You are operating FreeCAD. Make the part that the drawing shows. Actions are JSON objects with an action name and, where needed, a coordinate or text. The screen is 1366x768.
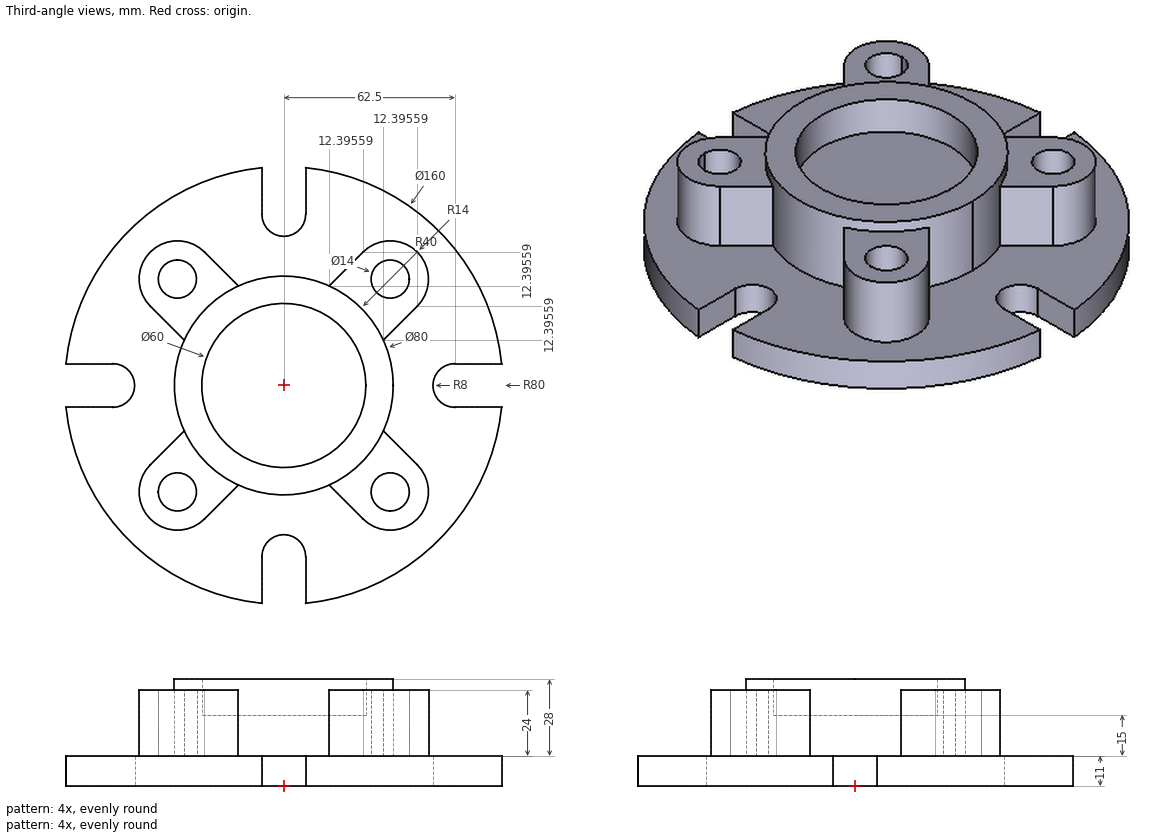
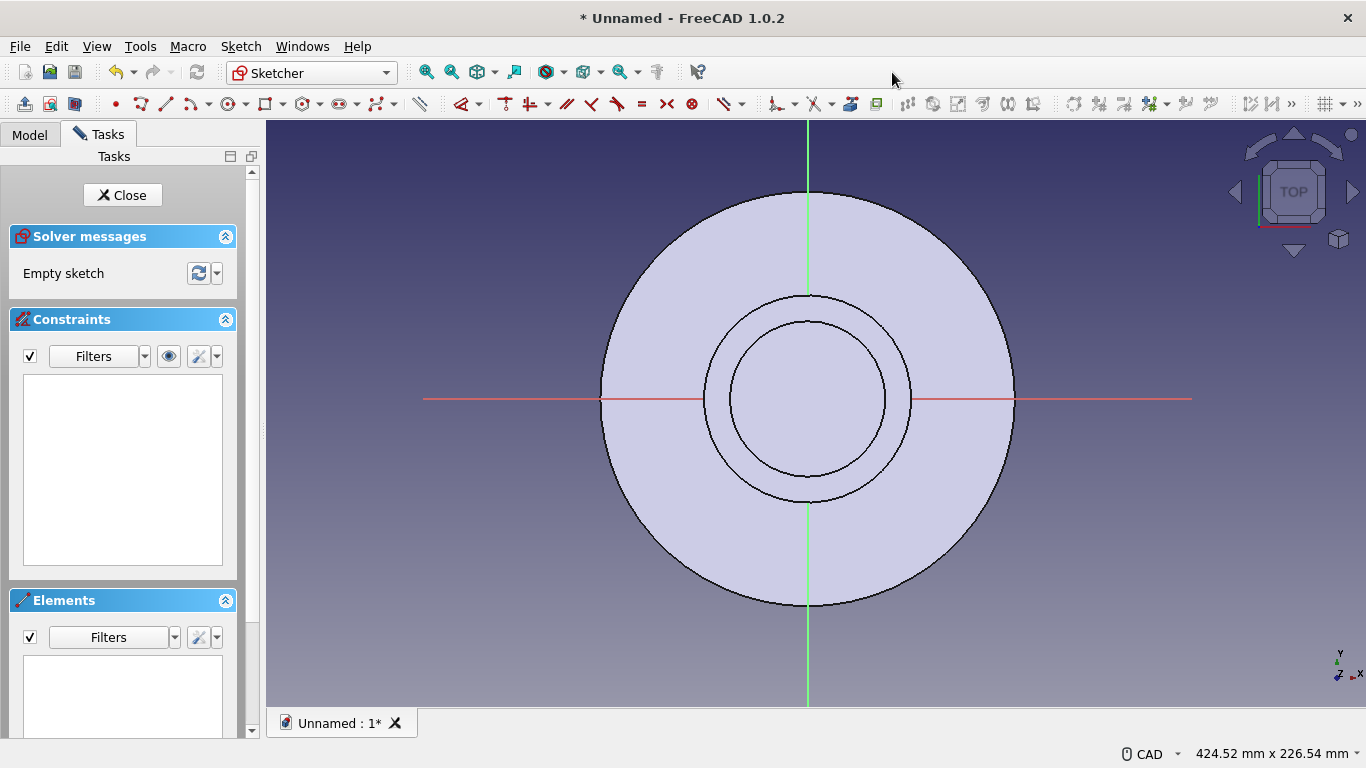
{"action": "key", "text": "q s"}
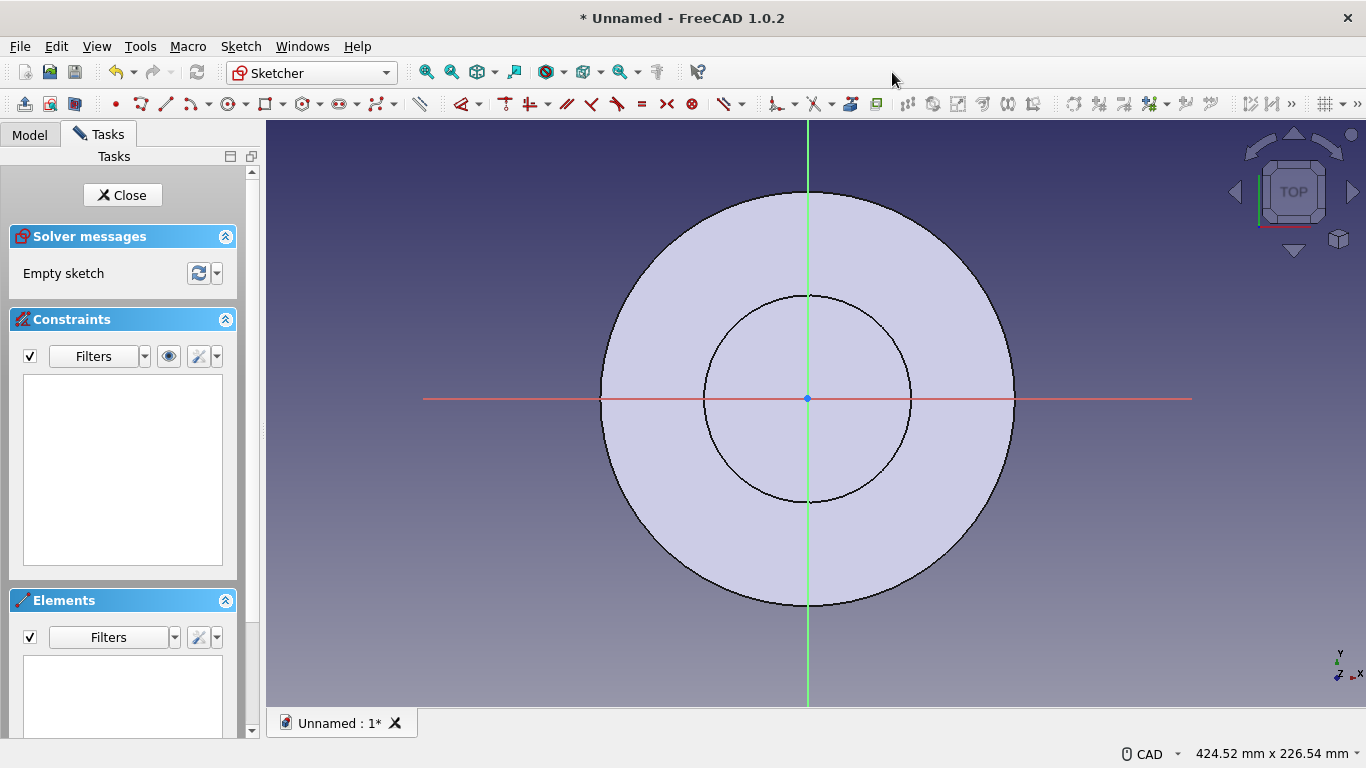
{"action": "scroll", "coordinate": [943, 291], "scroll_direction": "up", "scroll_amount": 5}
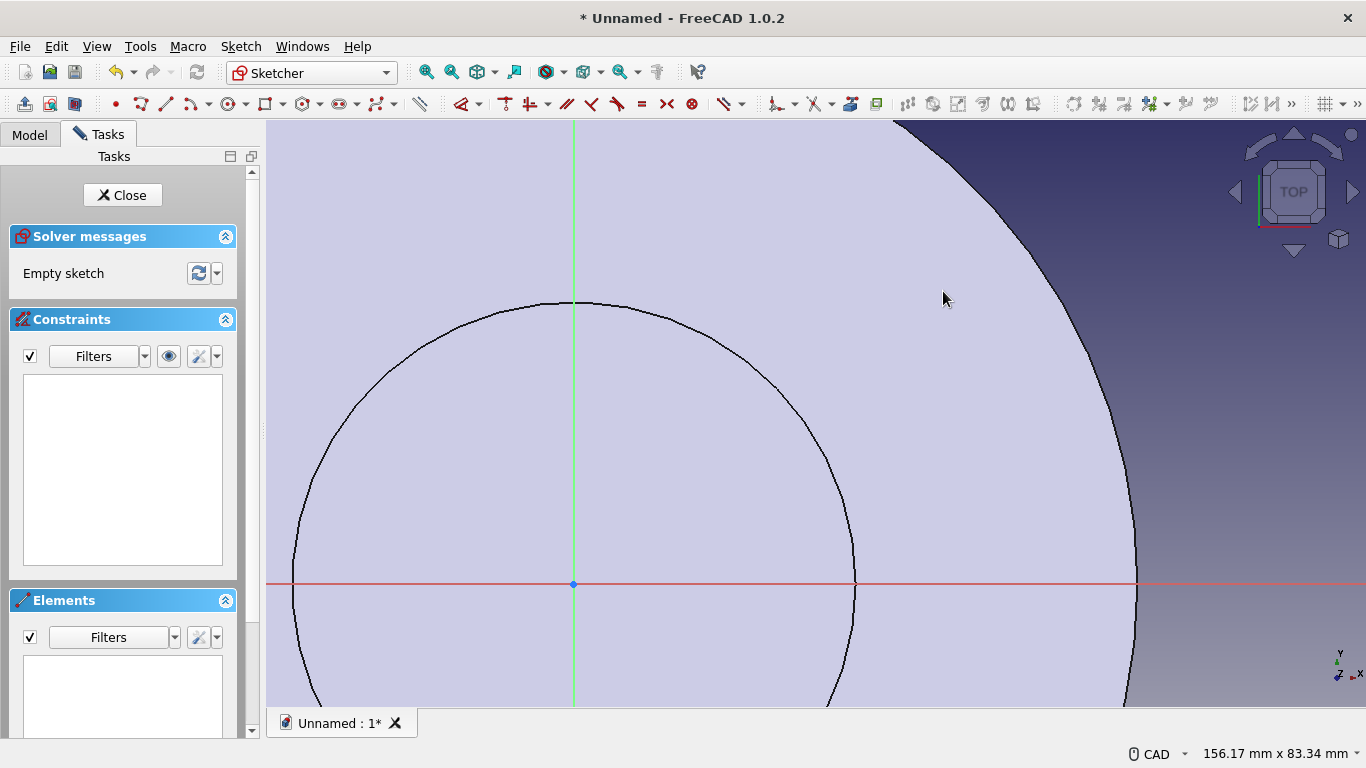
{"action": "key", "text": "g l"}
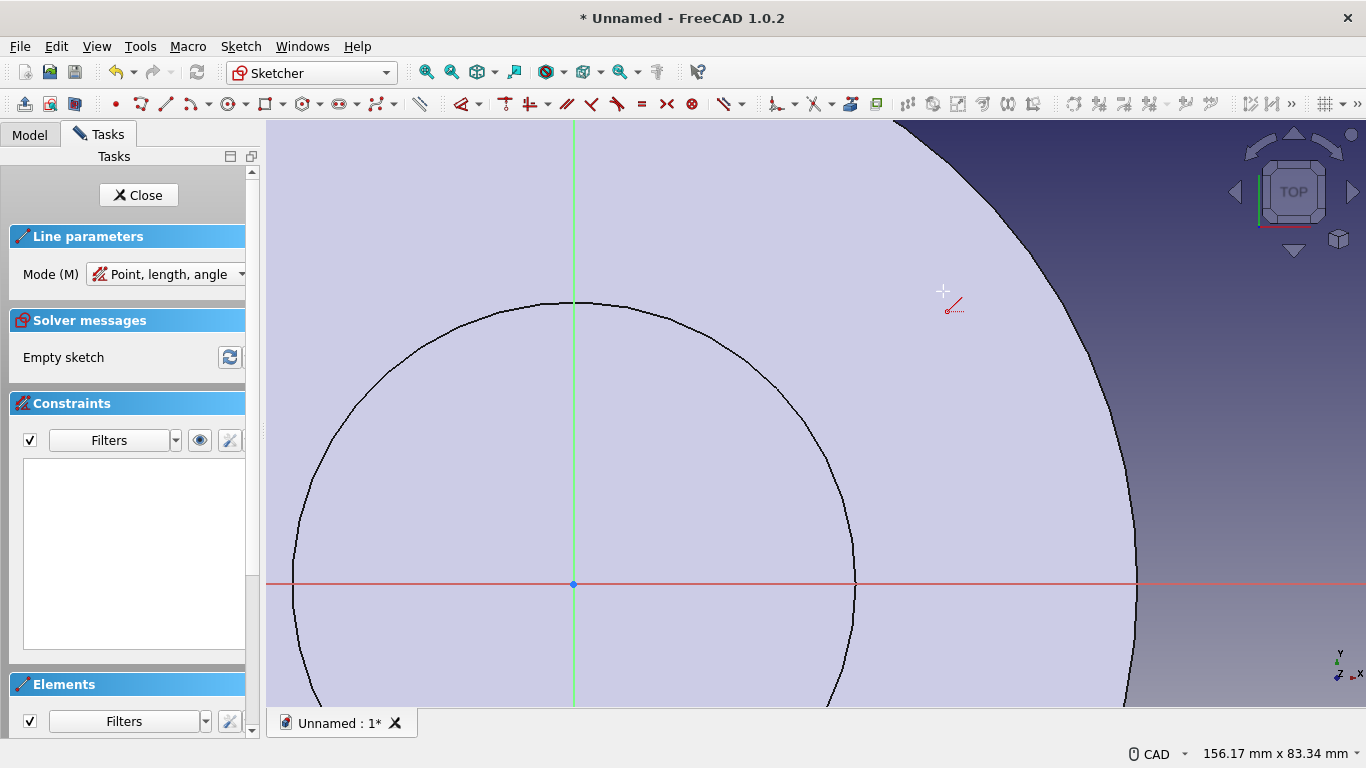
{"action": "left_click", "coordinate": [778, 240]}
{"action": "left_click", "coordinate": [691, 328]}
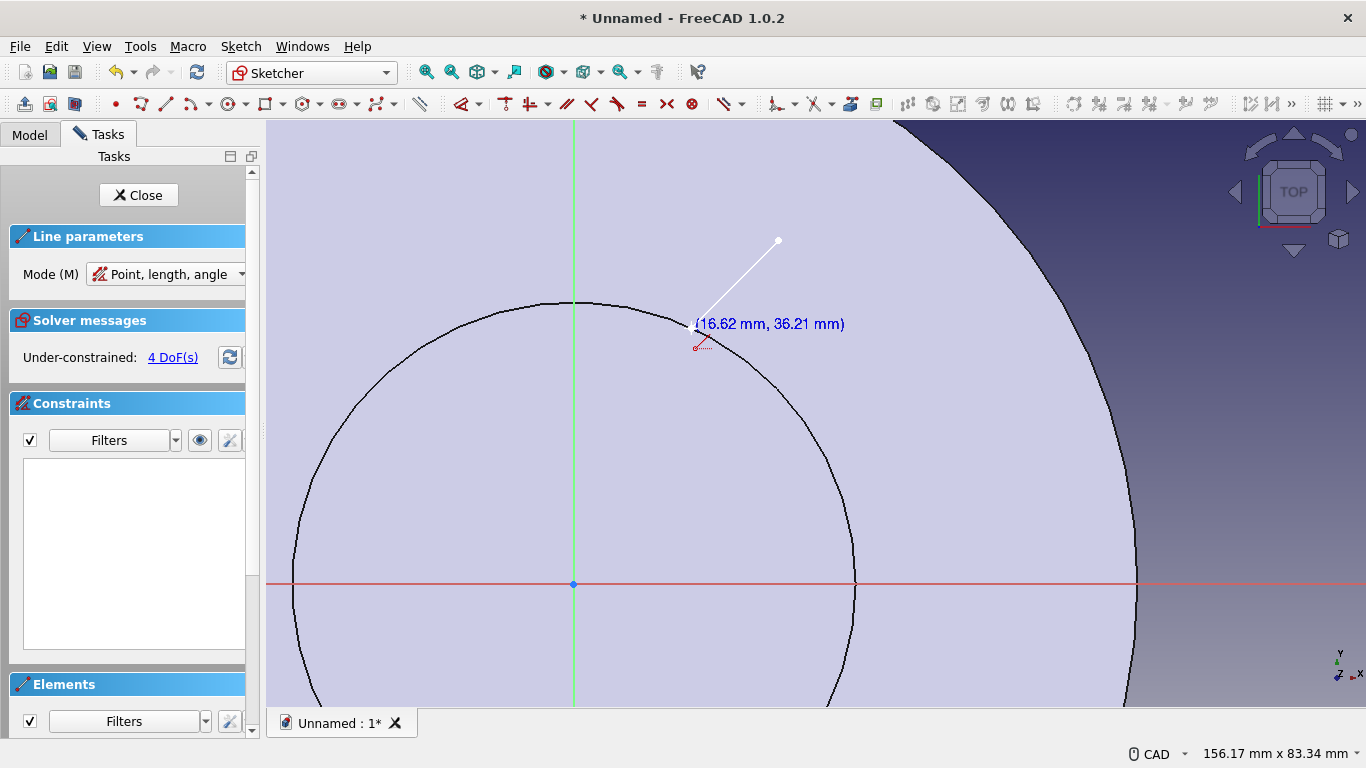
{"action": "left_click", "coordinate": [830, 467]}
{"action": "left_click", "coordinate": [918, 380]}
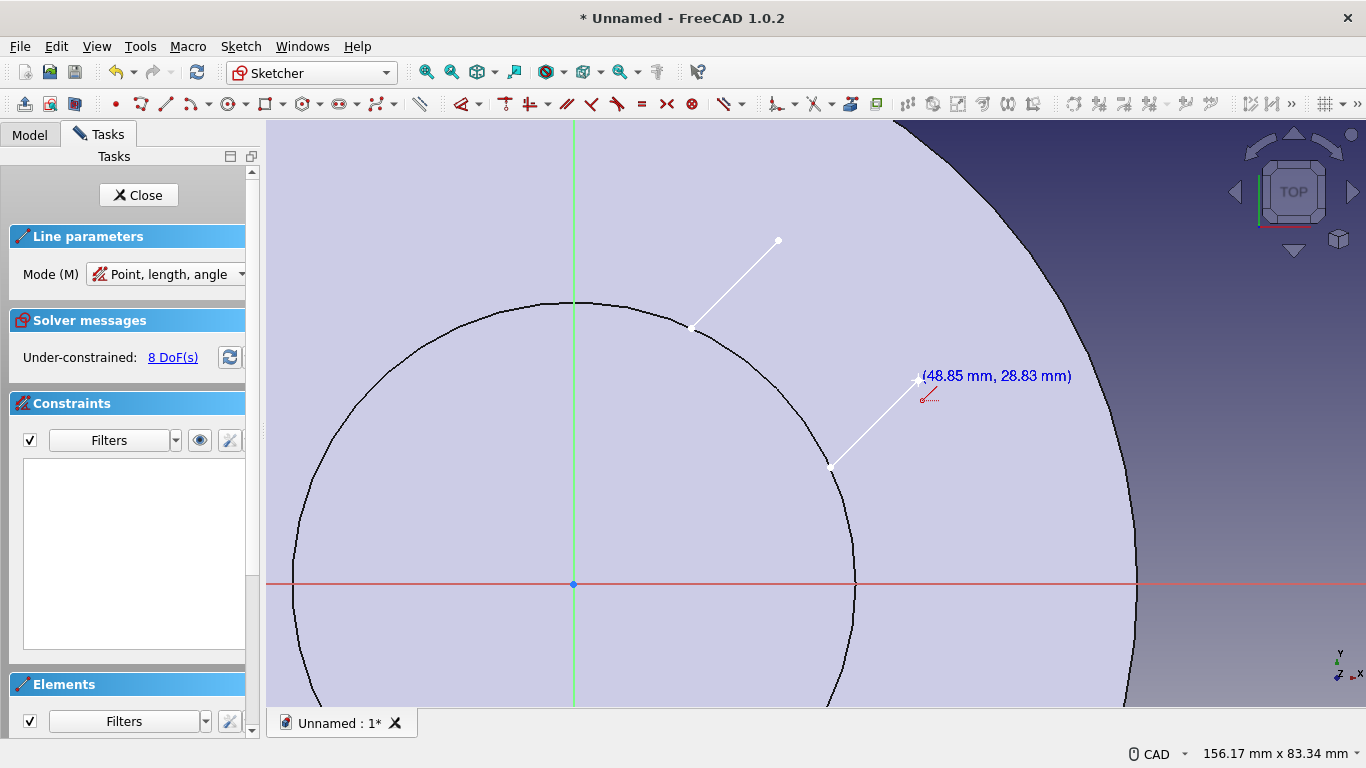
{"action": "key", "text": "g 3 a"}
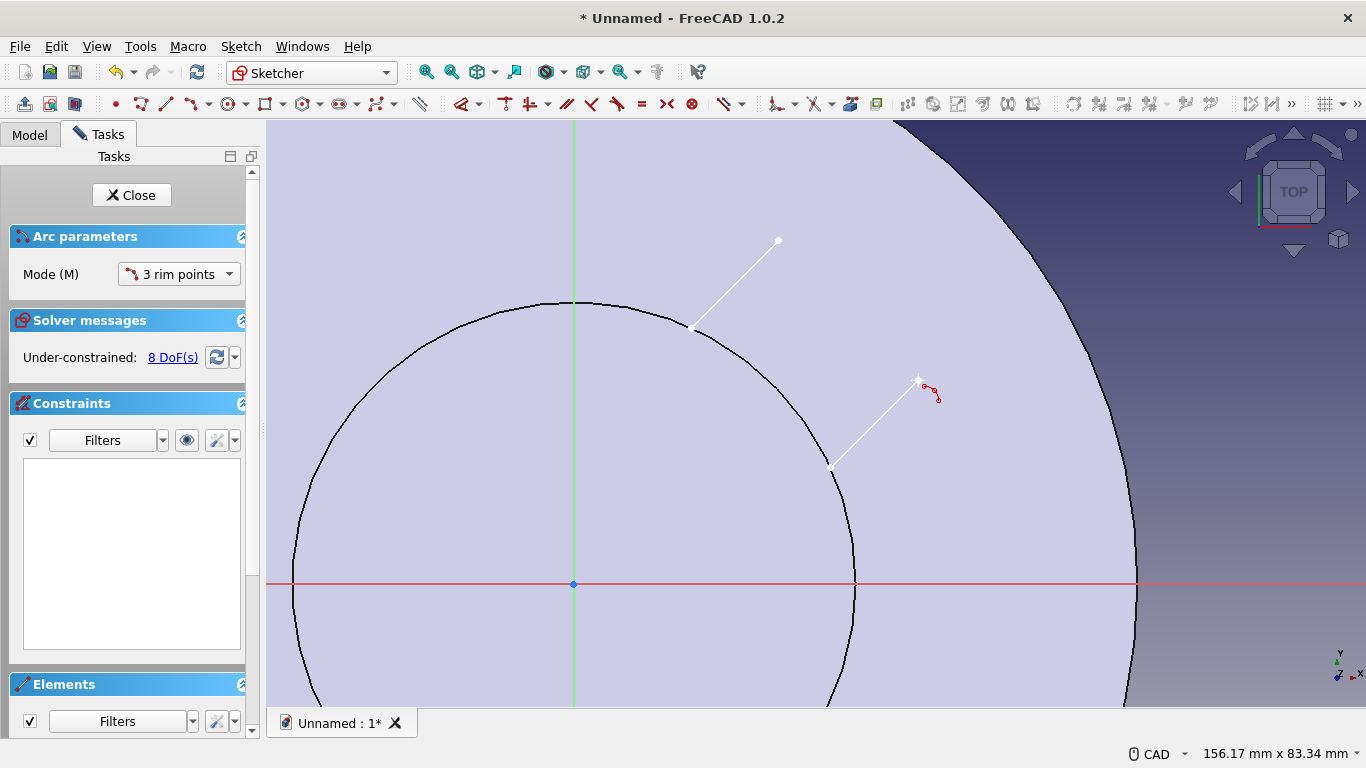
{"action": "left_click", "coordinate": [691, 329]}
{"action": "left_click", "coordinate": [830, 468]}
{"action": "left_click", "coordinate": [773, 385]}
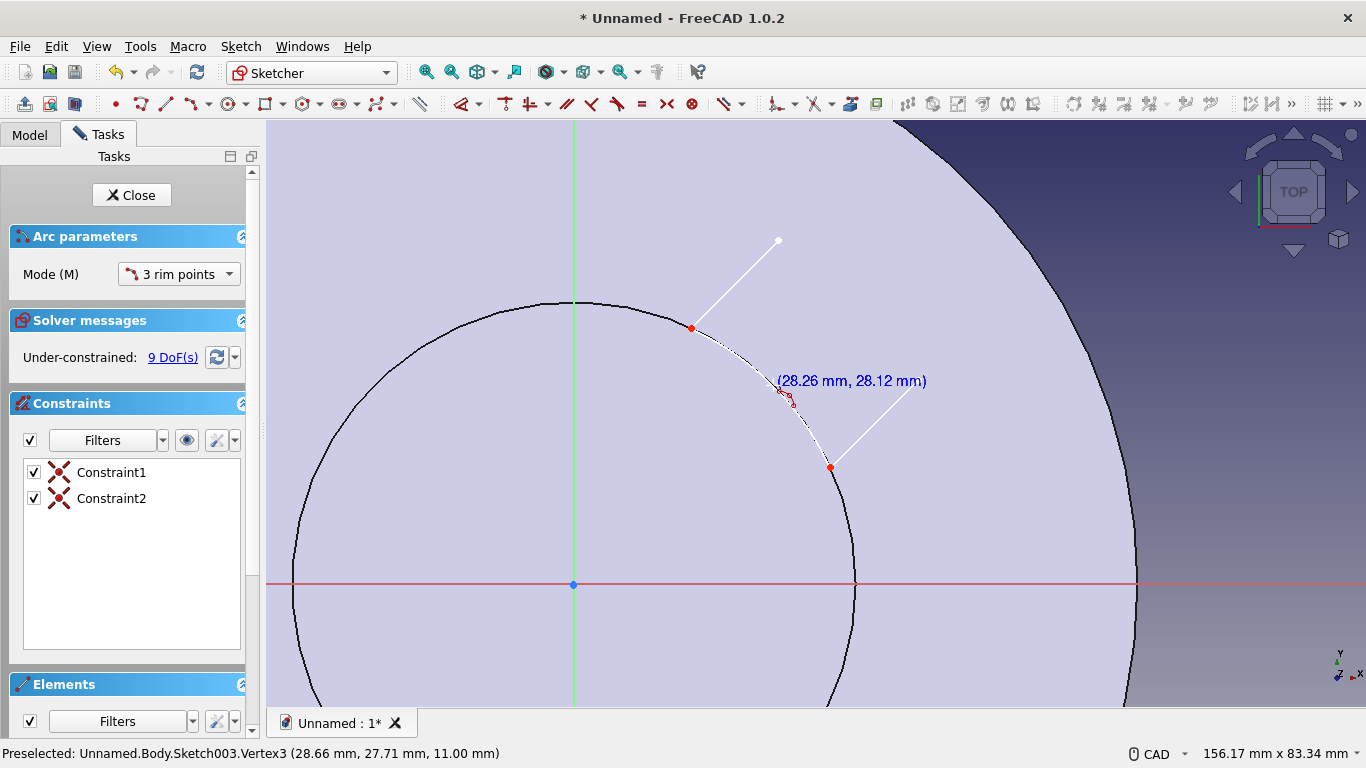
{"action": "left_click", "coordinate": [918, 381]}
{"action": "left_click", "coordinate": [778, 241]}
{"action": "left_click", "coordinate": [918, 240]}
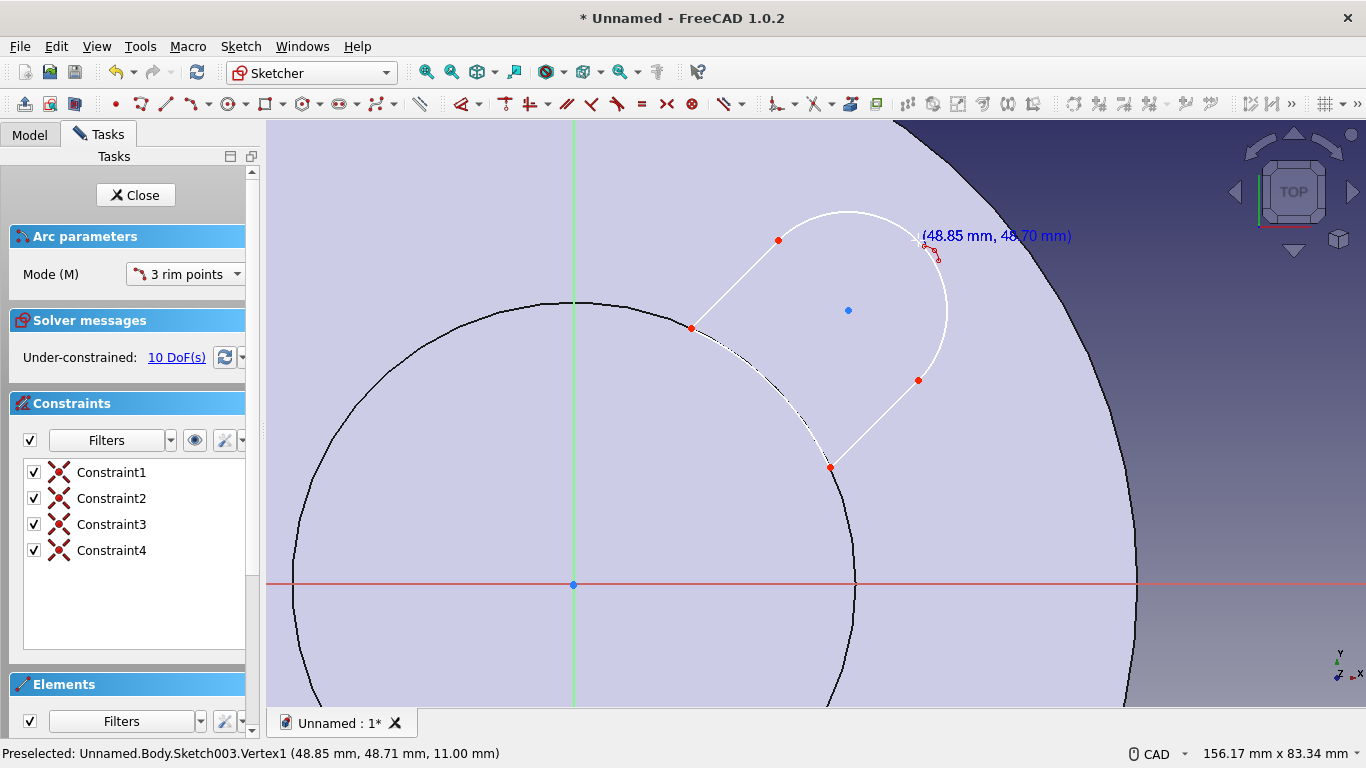
{"action": "key", "text": "g c"}